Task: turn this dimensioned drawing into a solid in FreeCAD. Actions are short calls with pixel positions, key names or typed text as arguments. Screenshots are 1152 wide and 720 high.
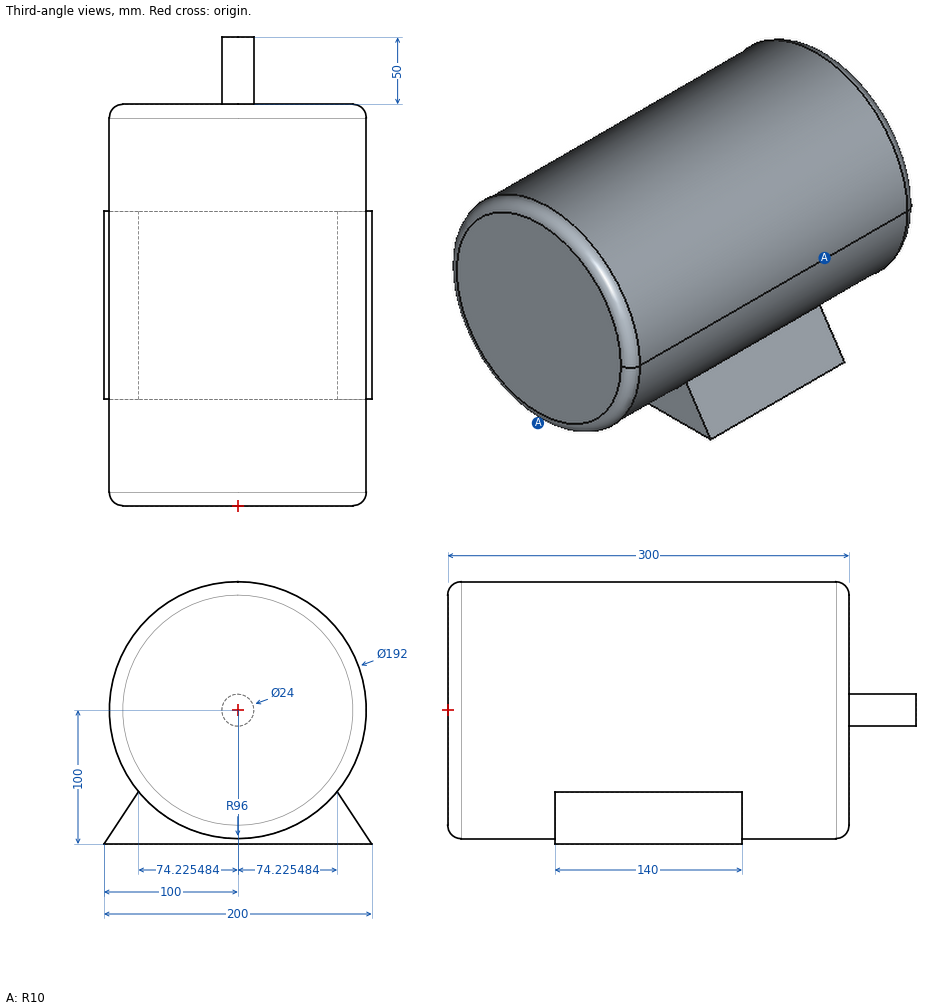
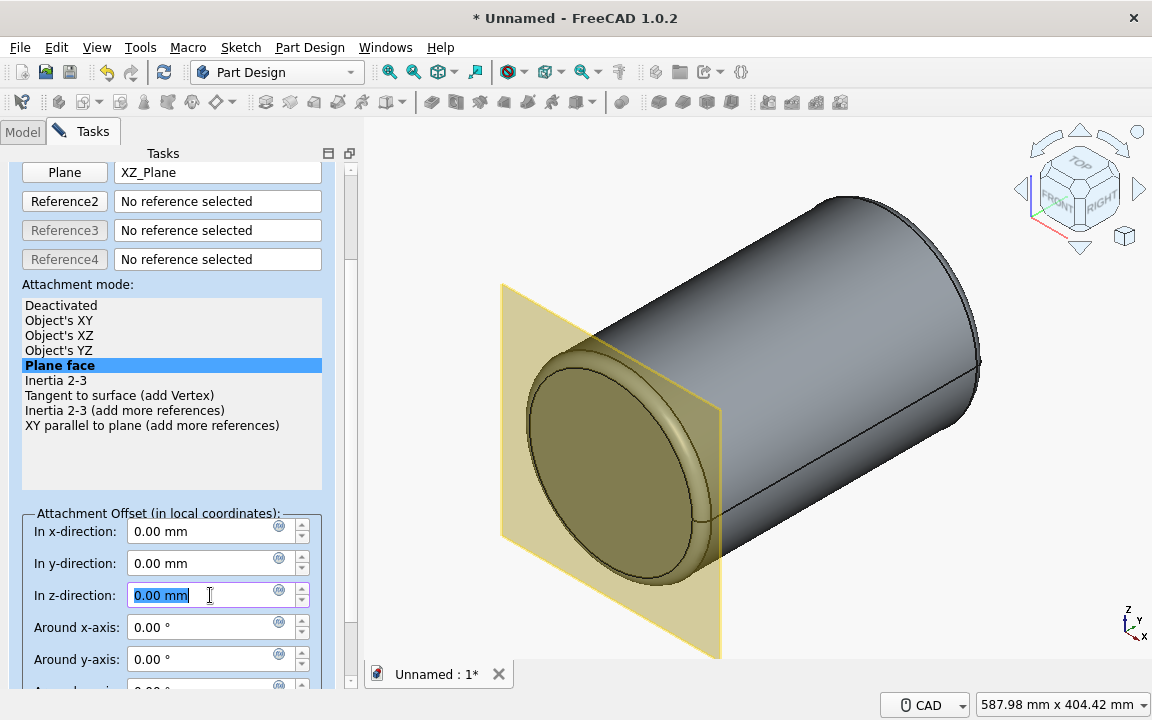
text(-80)
key(Tab)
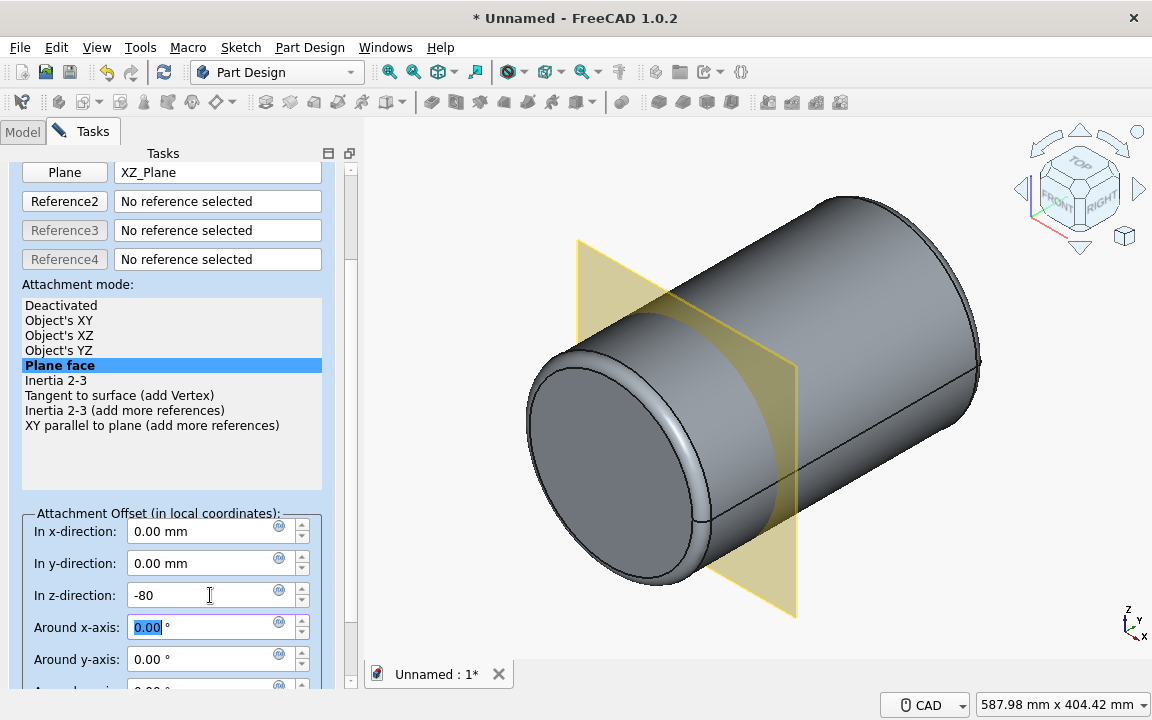
scroll(351, 426, up, 3)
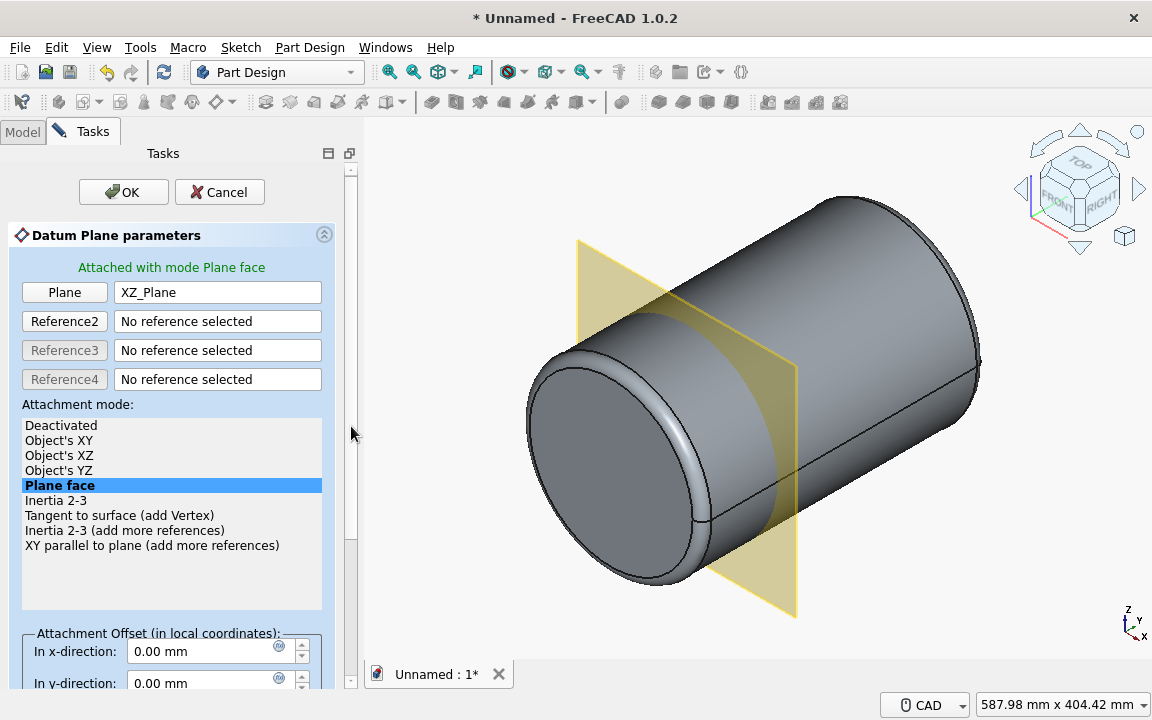
click(124, 192)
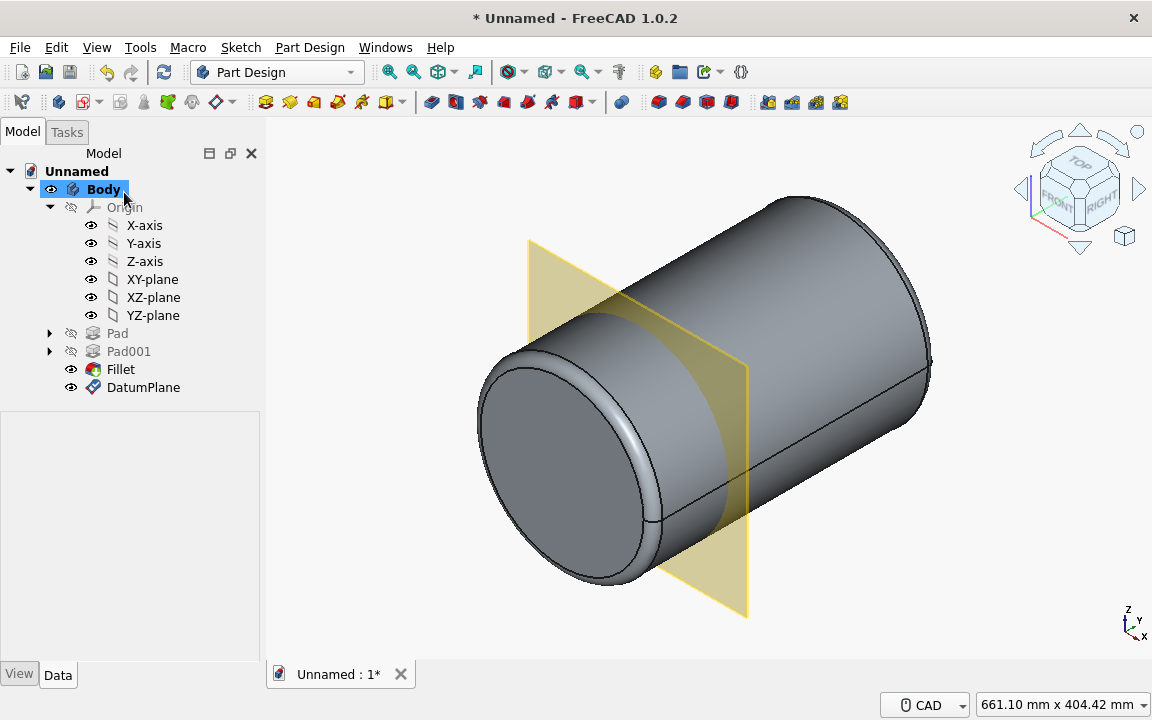
click(116, 387)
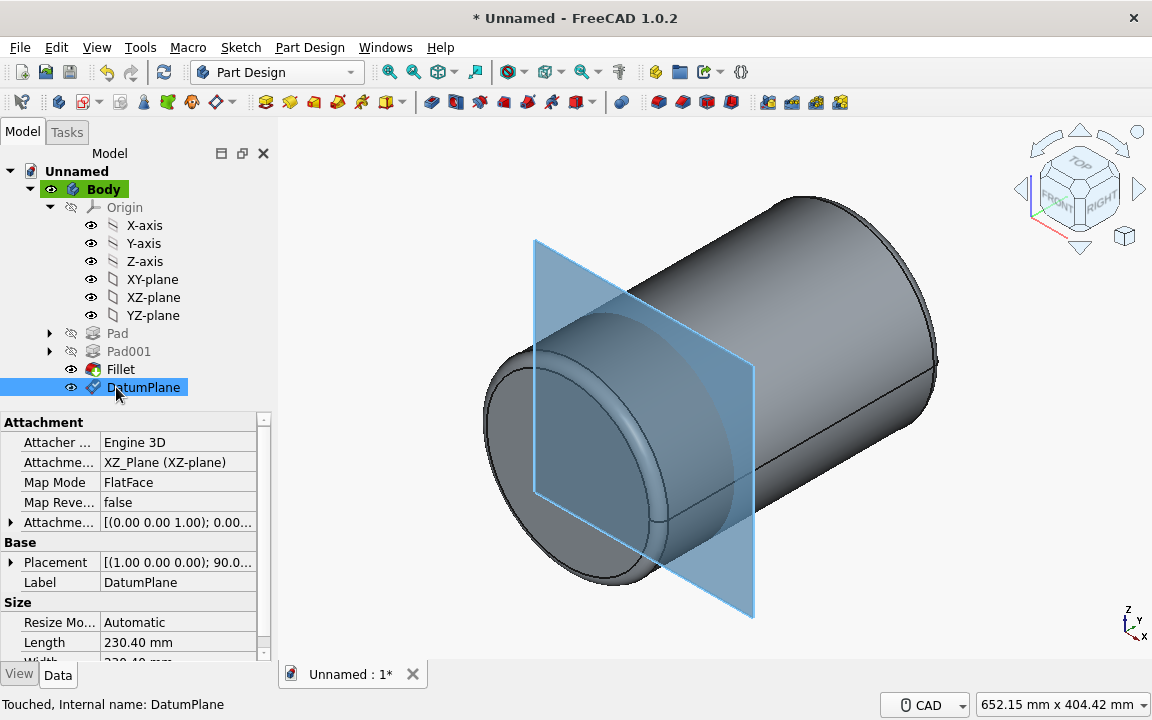
click(84, 102)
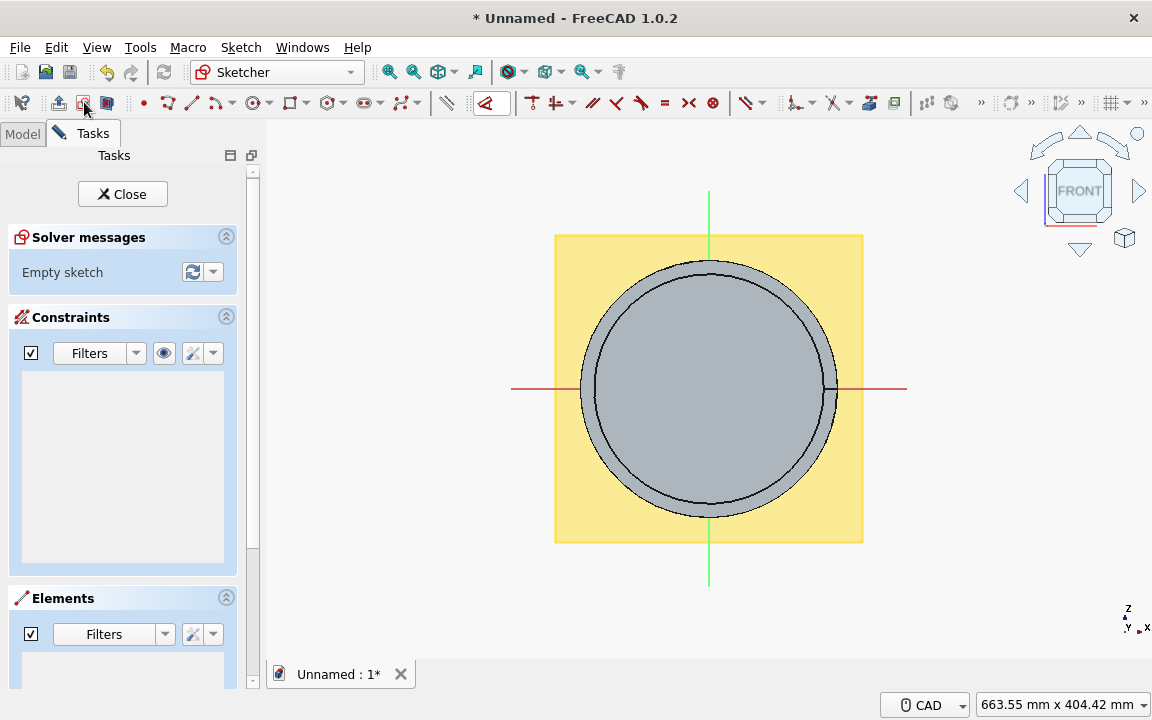
click(108, 104)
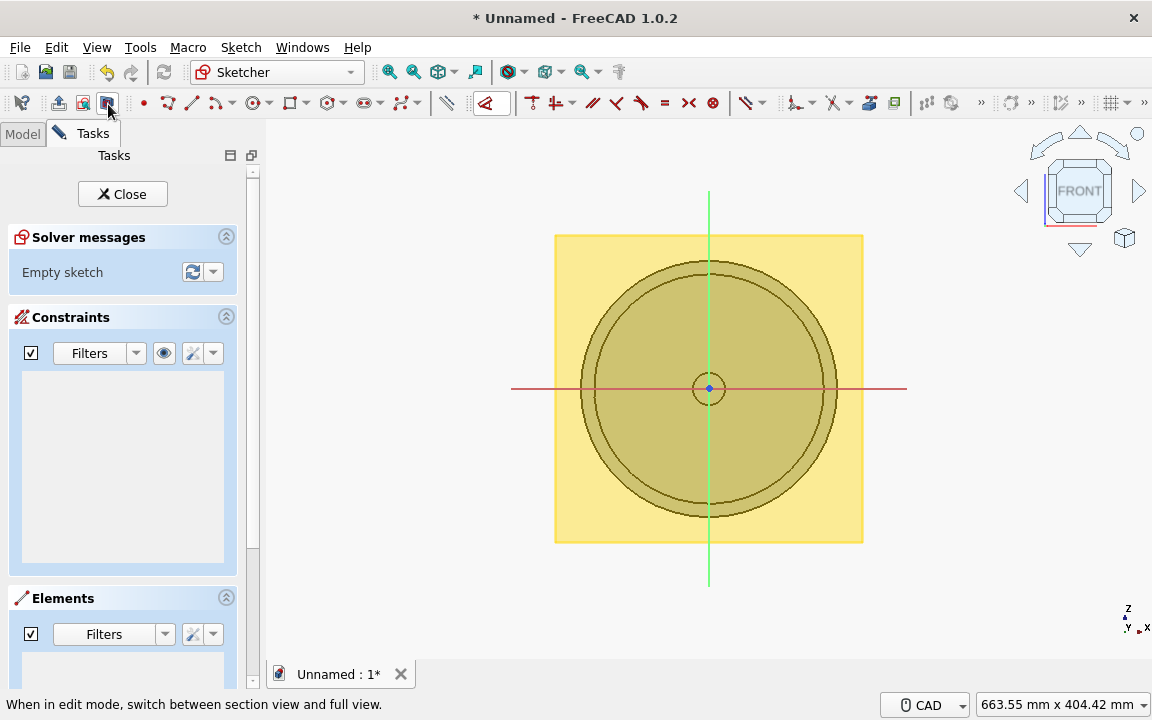
scroll(792, 537, up, 3)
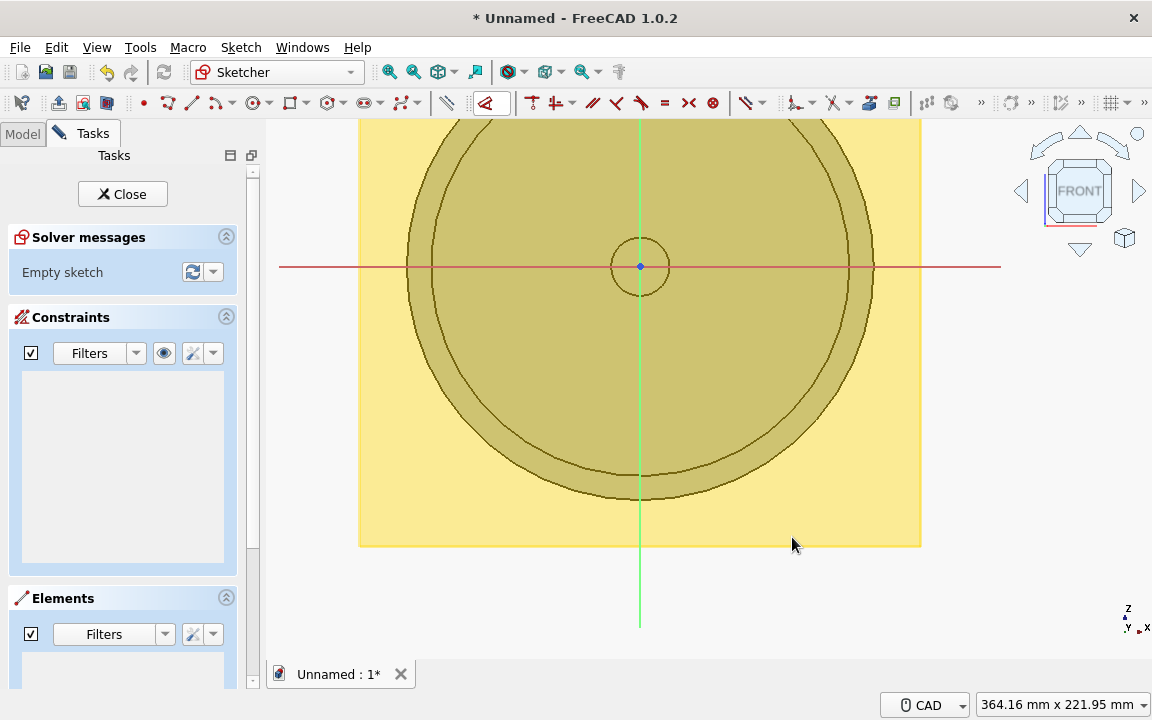
key(g)
key(m)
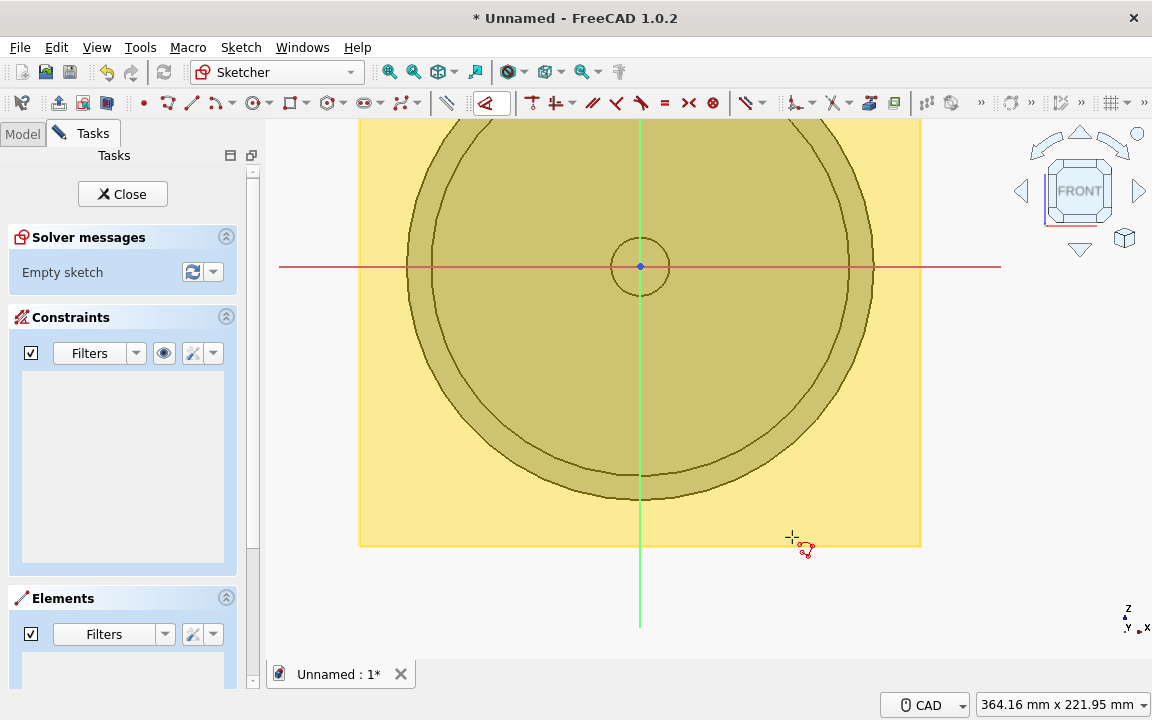
click(460, 415)
click(397, 510)
click(884, 510)
click(821, 415)
right_click(821, 415)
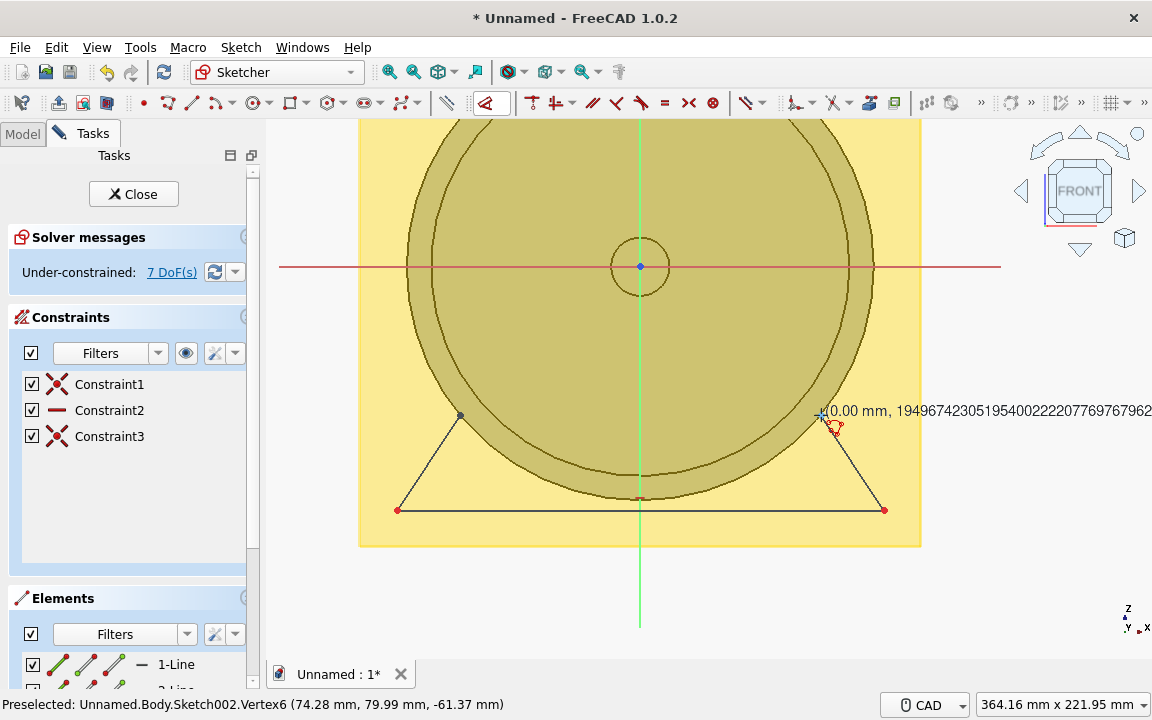
click(234, 104)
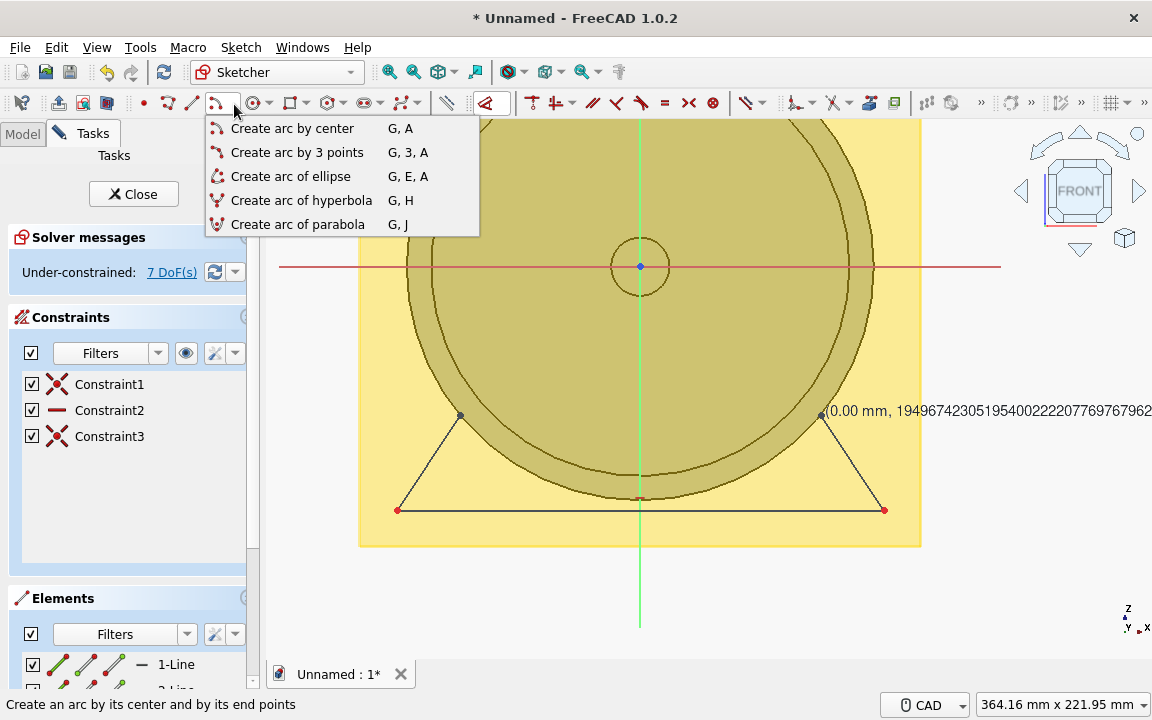
click(342, 152)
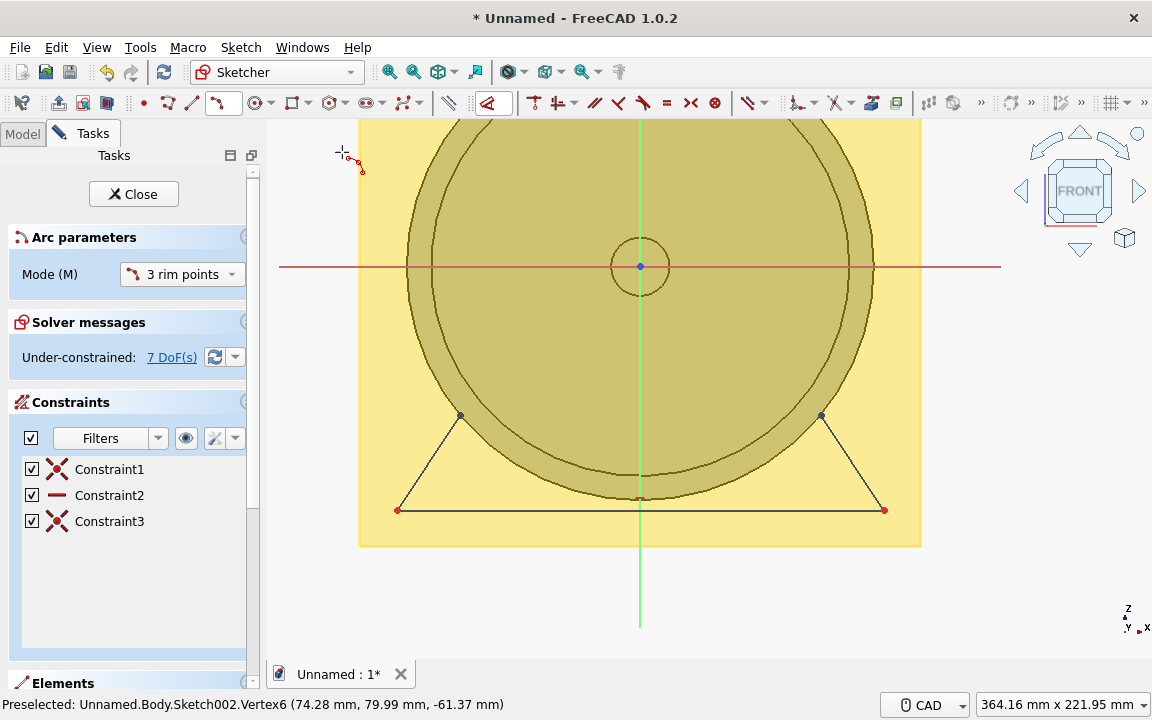
click(821, 416)
click(460, 416)
click(559, 486)
key(Escape)